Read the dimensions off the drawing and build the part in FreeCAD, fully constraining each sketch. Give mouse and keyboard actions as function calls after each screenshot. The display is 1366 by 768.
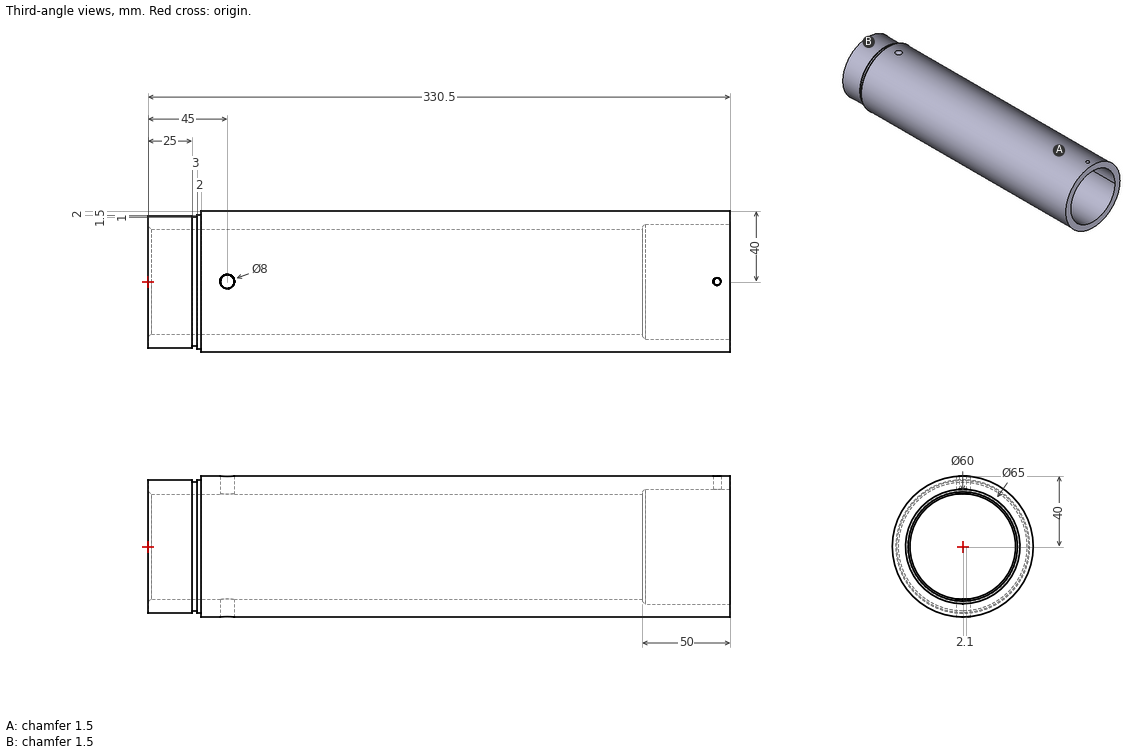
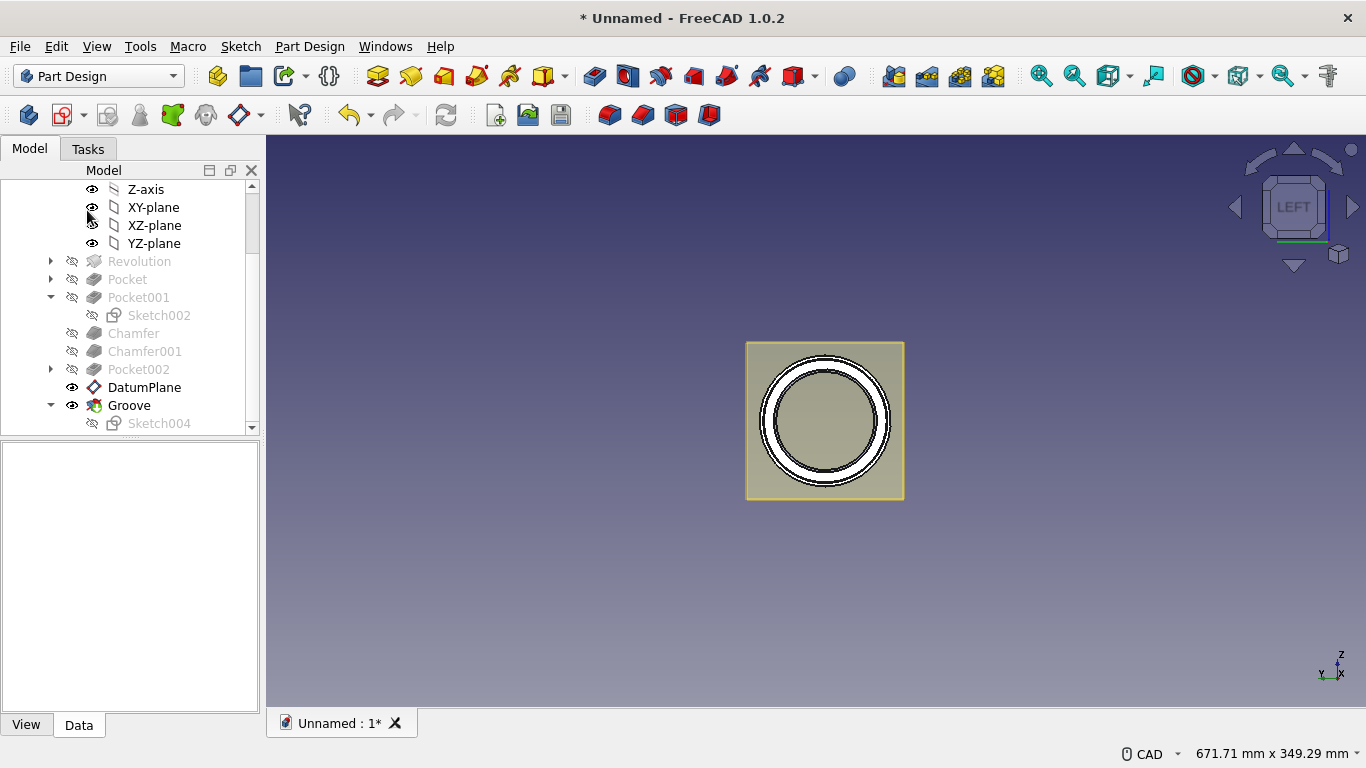
click(117, 387)
key(space)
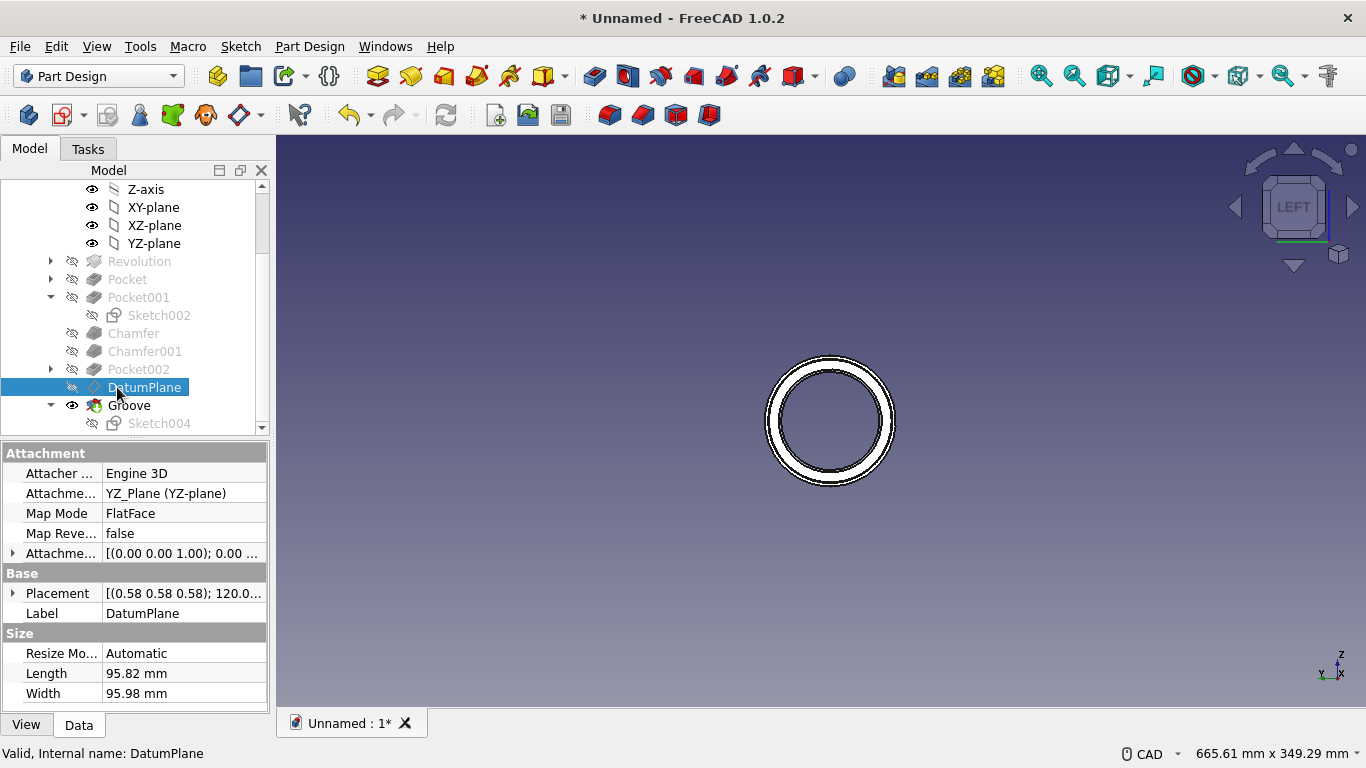
key(0)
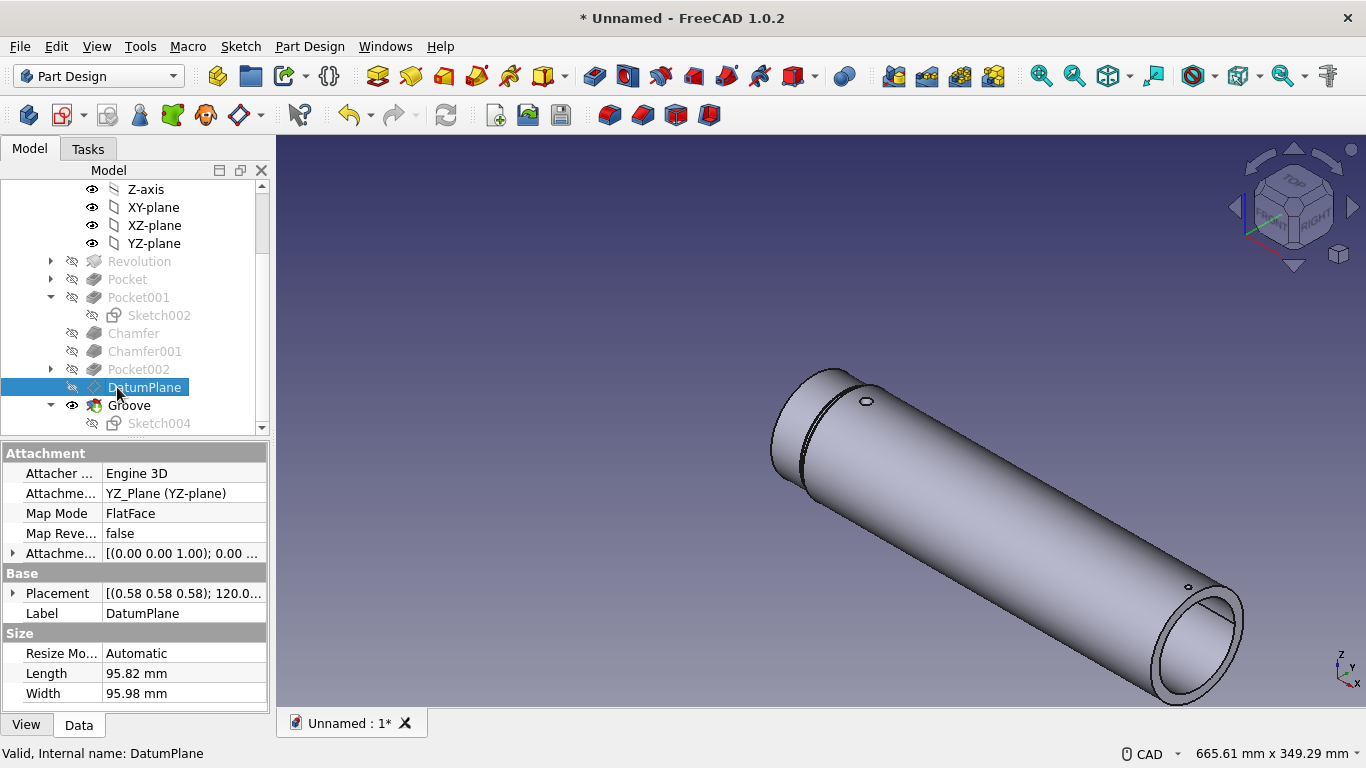
click(1042, 76)